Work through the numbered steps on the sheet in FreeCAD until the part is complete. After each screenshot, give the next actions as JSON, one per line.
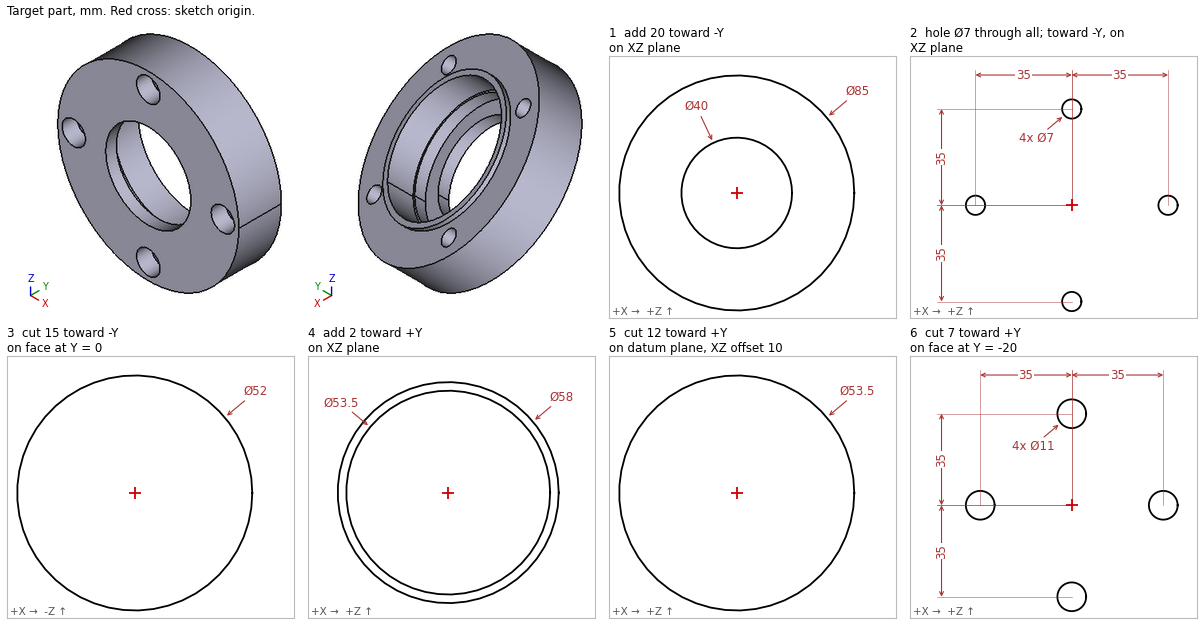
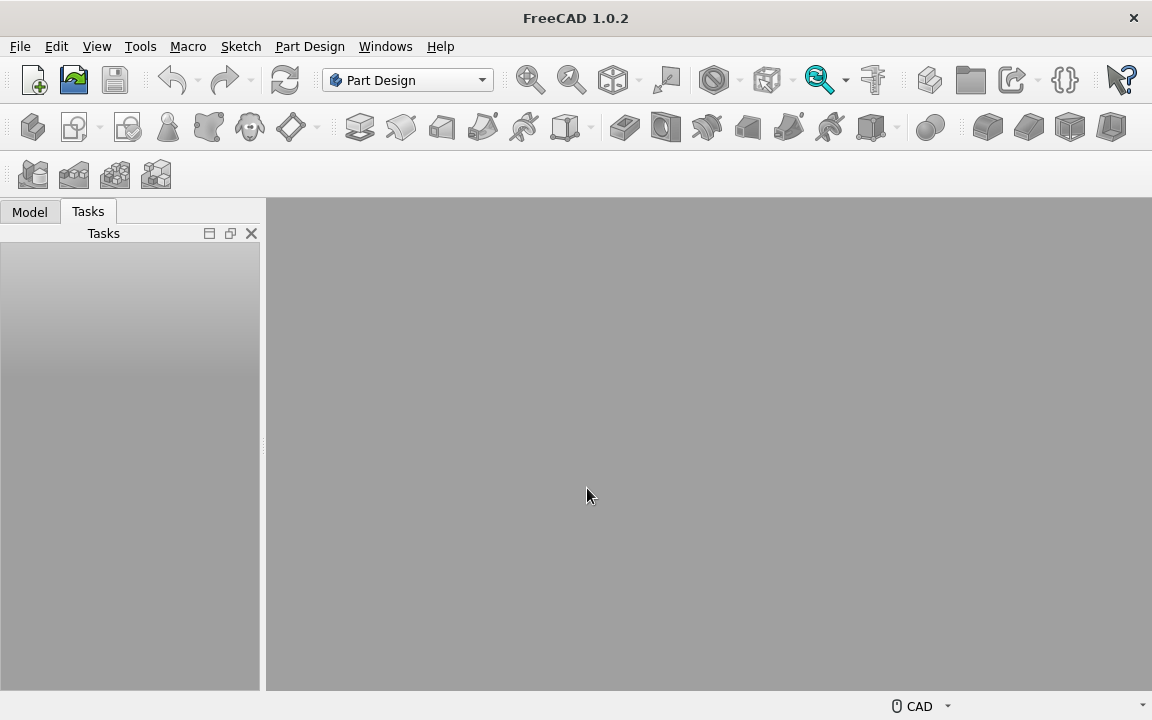
{"action": "key", "text": "ctrl+n"}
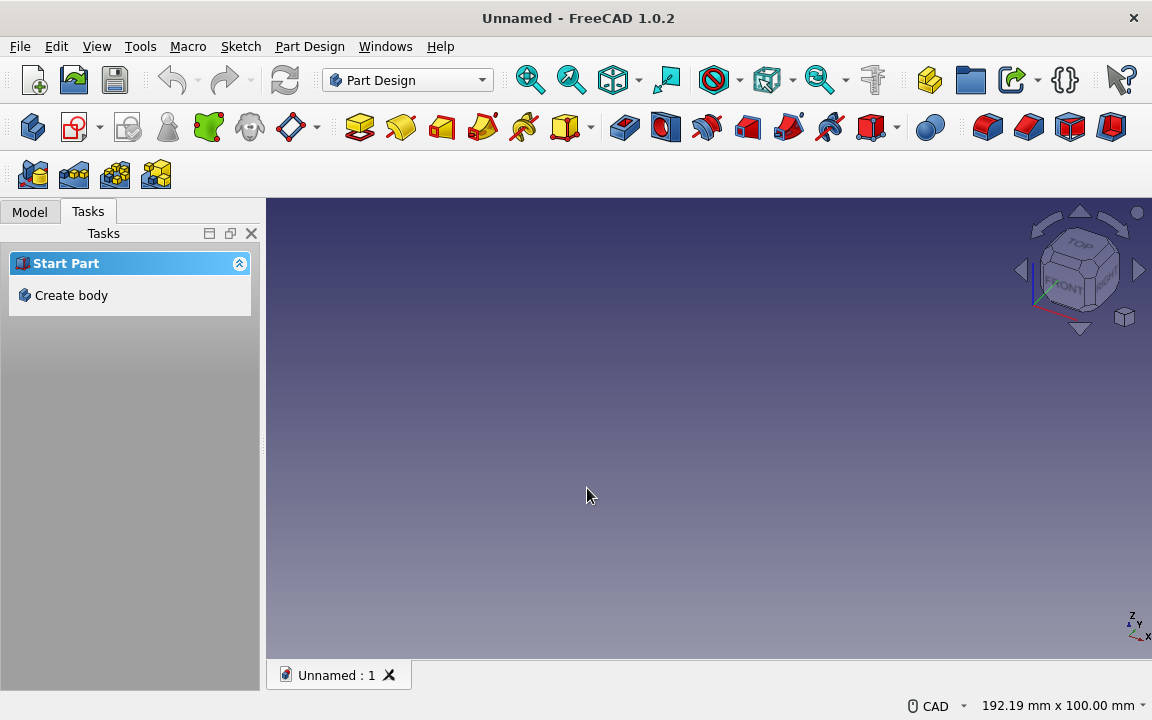
{"action": "left_click", "coordinate": [74, 128]}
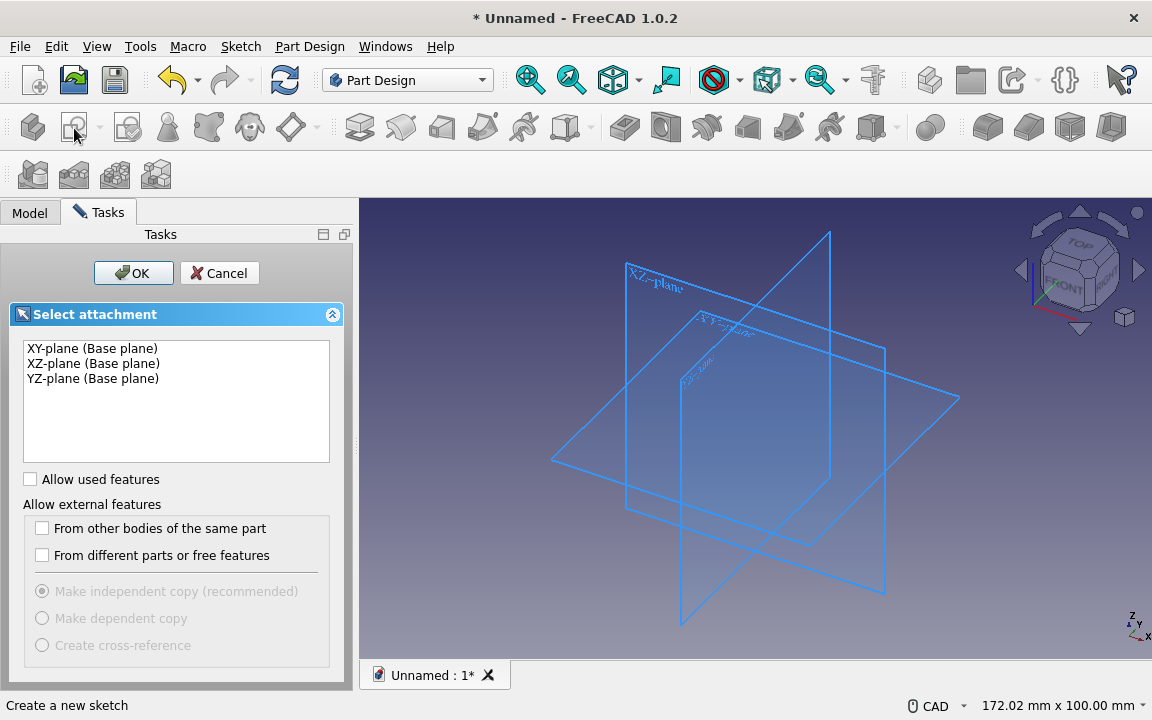
{"action": "left_click", "coordinate": [84, 364]}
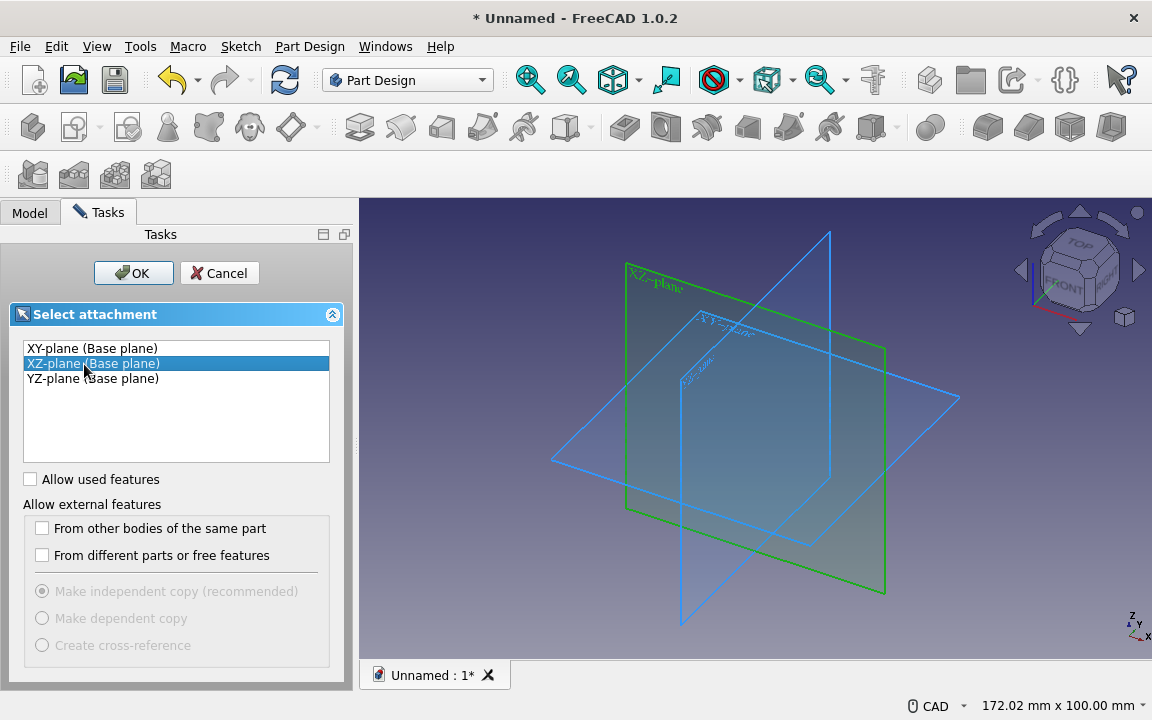
{"action": "left_click", "coordinate": [134, 273]}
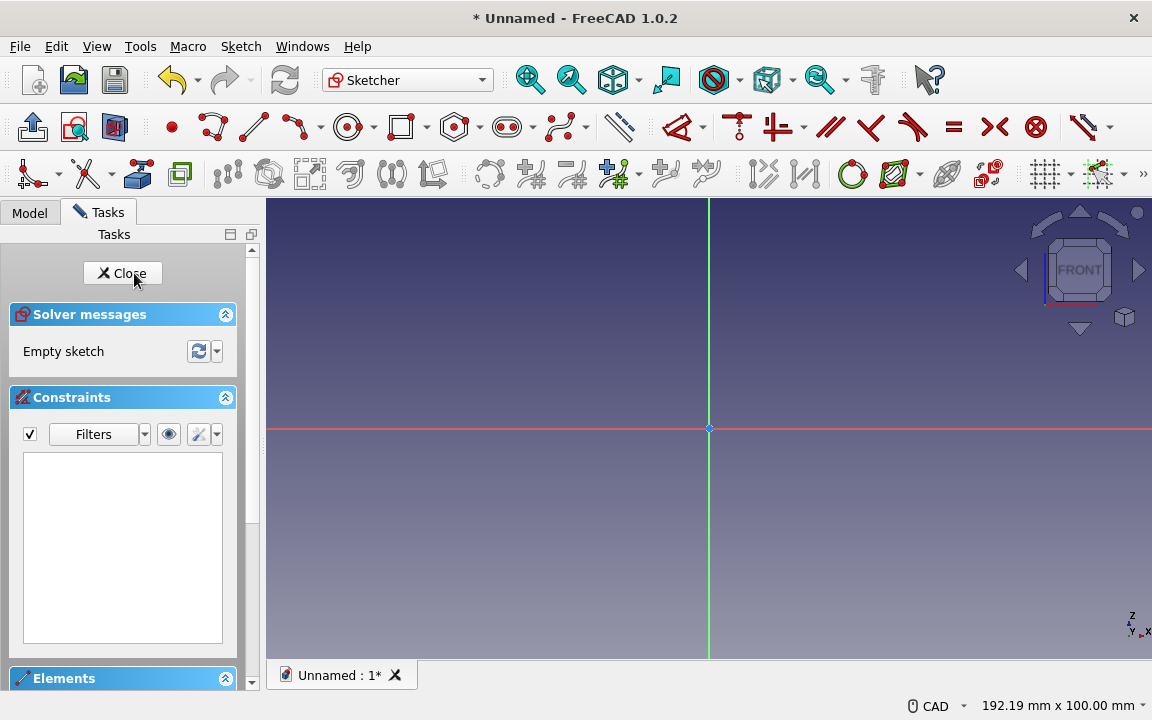
{"action": "scroll", "coordinate": [501, 429], "scroll_direction": "down", "scroll_amount": 2}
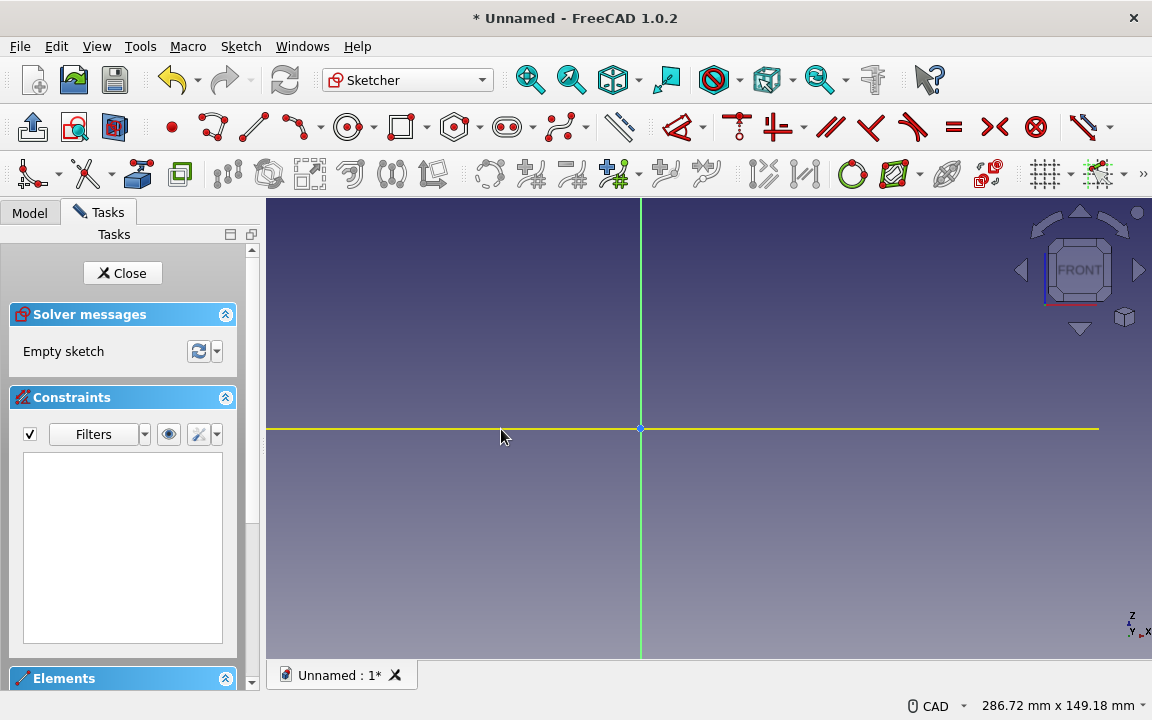
{"action": "key", "text": "g c"}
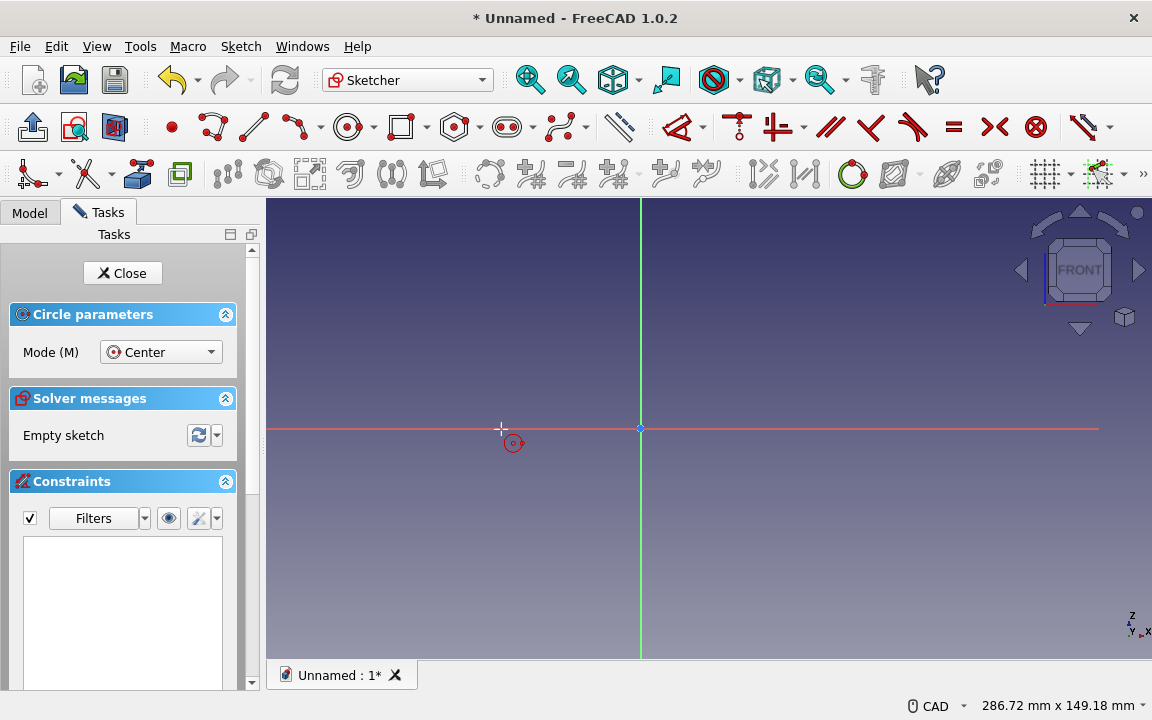
{"action": "left_click", "coordinate": [641, 429]}
{"action": "mouse_move", "coordinate": [733, 336]}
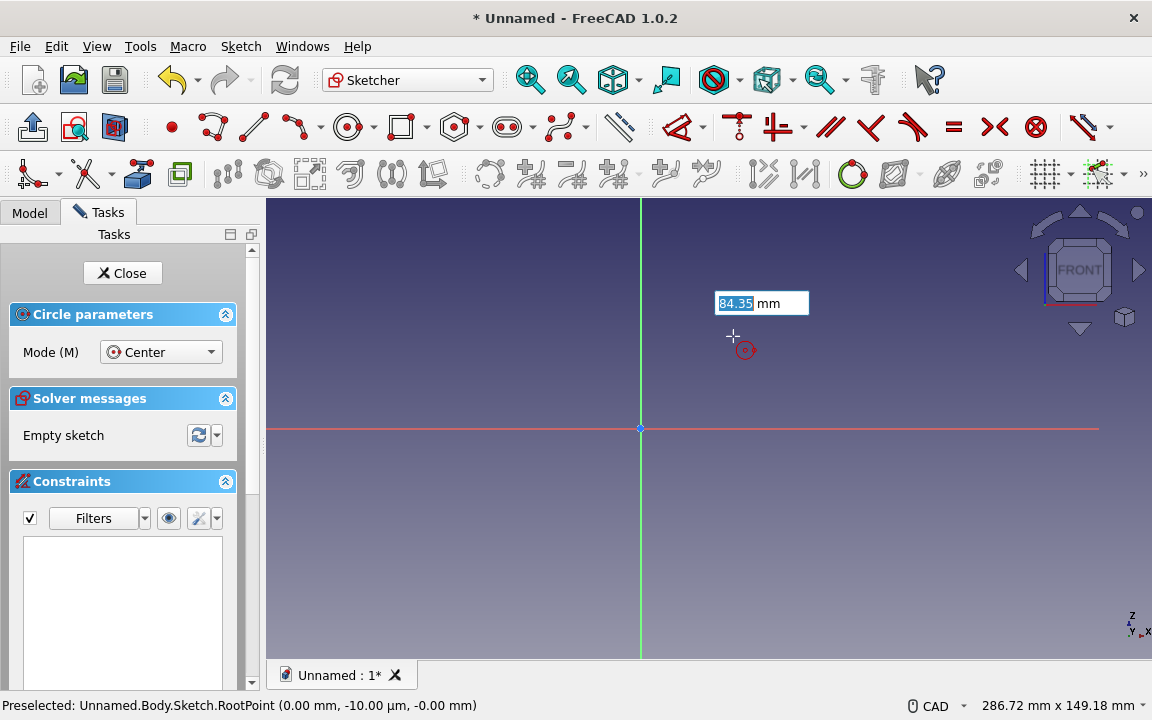
{"action": "type", "text": "85"}
{"action": "key", "text": "Return"}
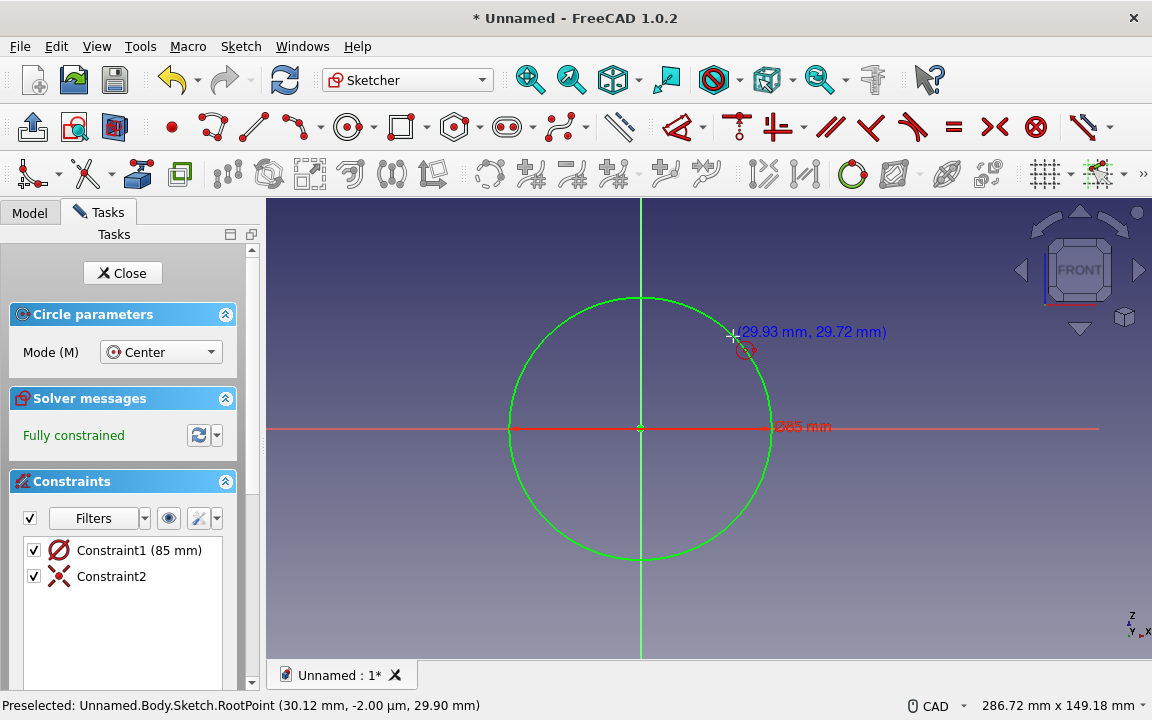
{"action": "left_click", "coordinate": [641, 429]}
{"action": "mouse_move", "coordinate": [684, 385]}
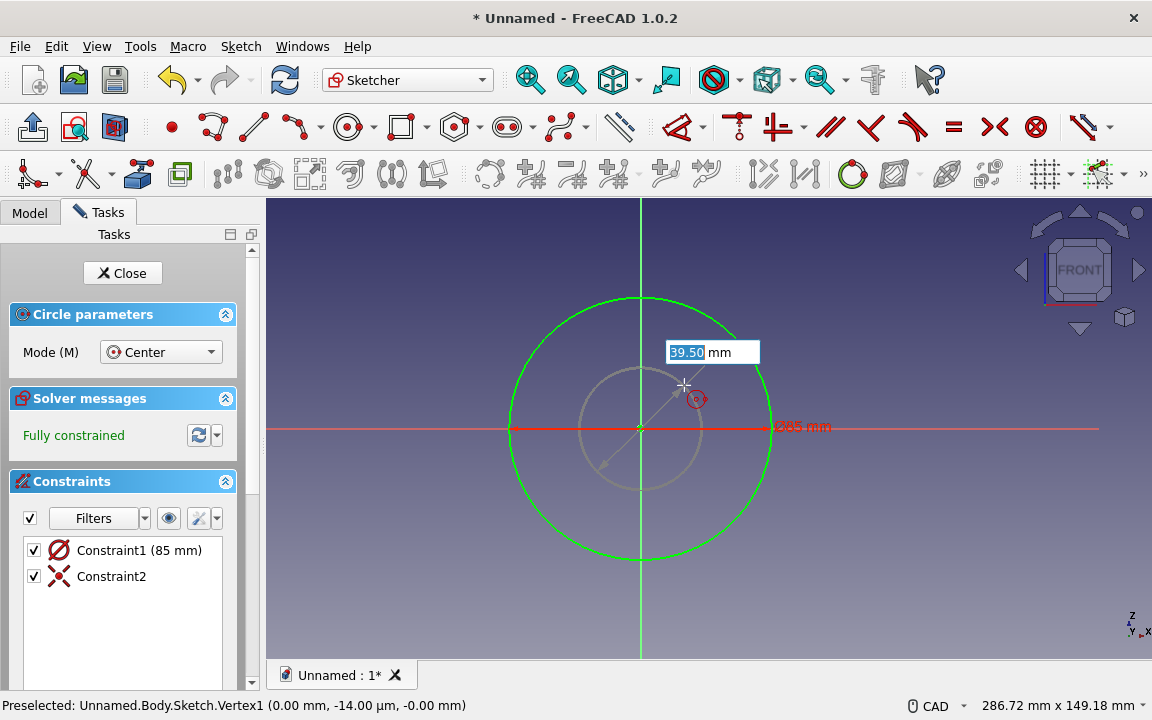
{"action": "type", "text": "40"}
{"action": "key", "text": "Return"}
{"action": "key", "text": "Escape"}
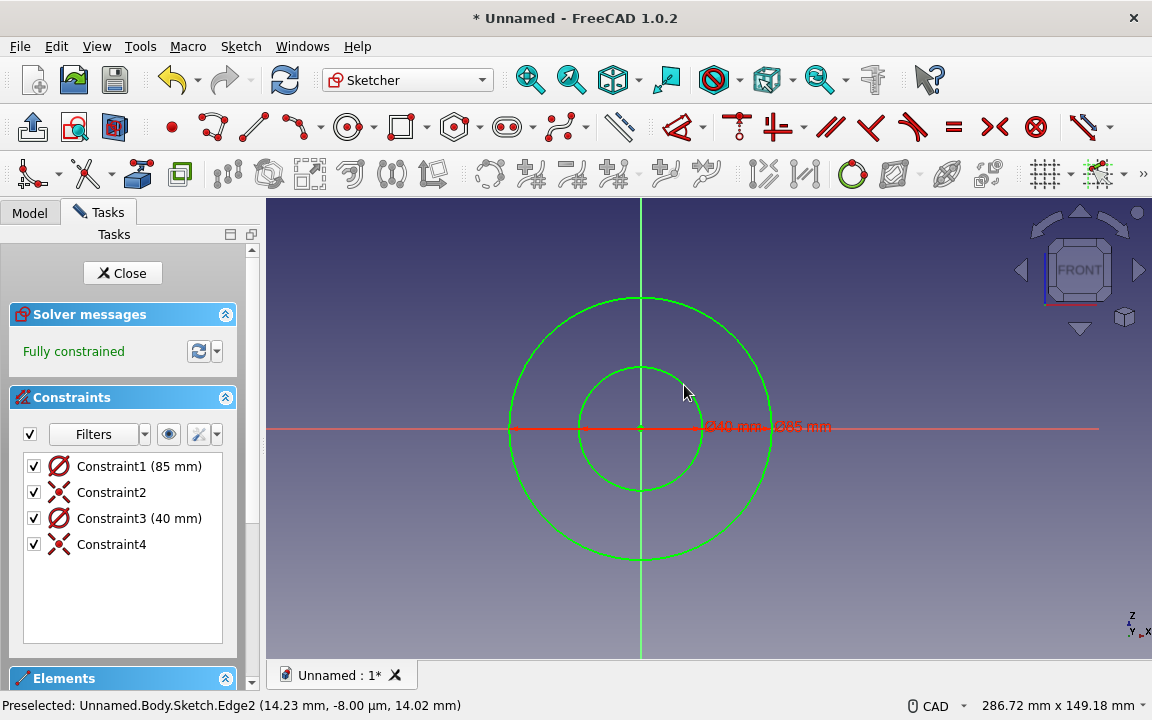
{"action": "left_click", "coordinate": [123, 273]}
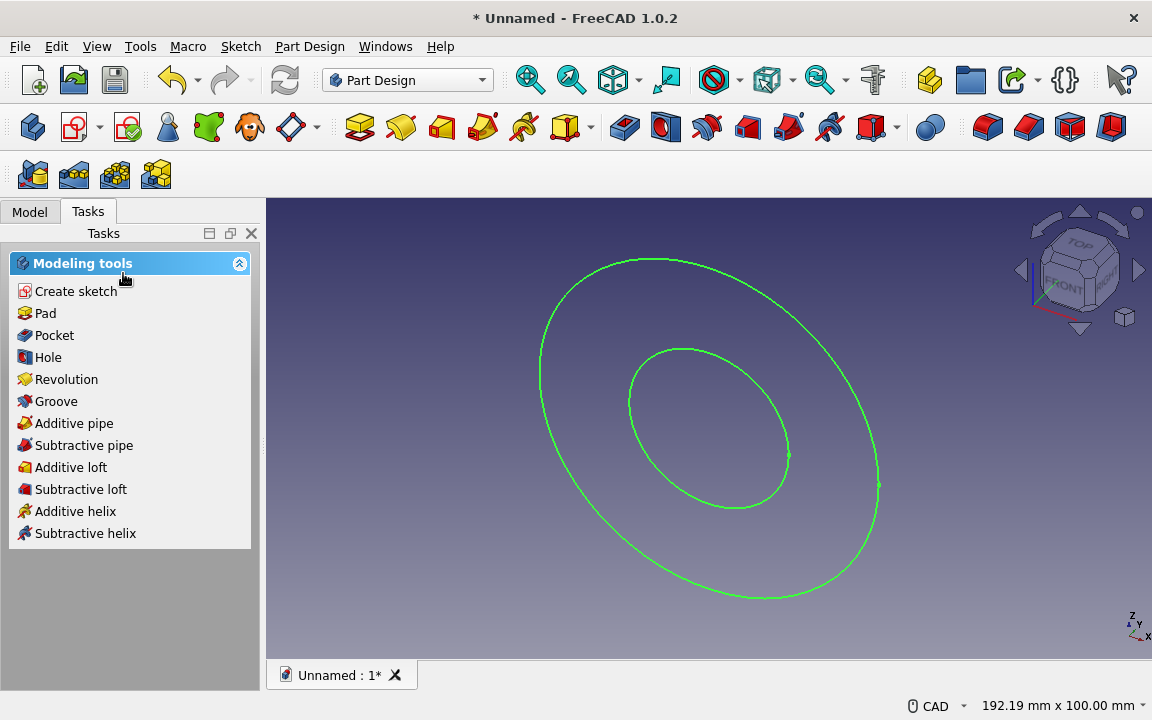
{"action": "left_click", "coordinate": [360, 128]}